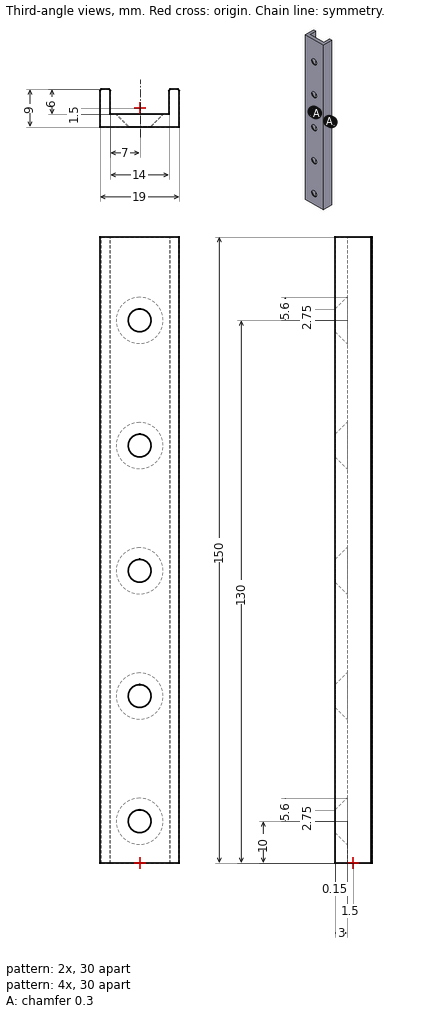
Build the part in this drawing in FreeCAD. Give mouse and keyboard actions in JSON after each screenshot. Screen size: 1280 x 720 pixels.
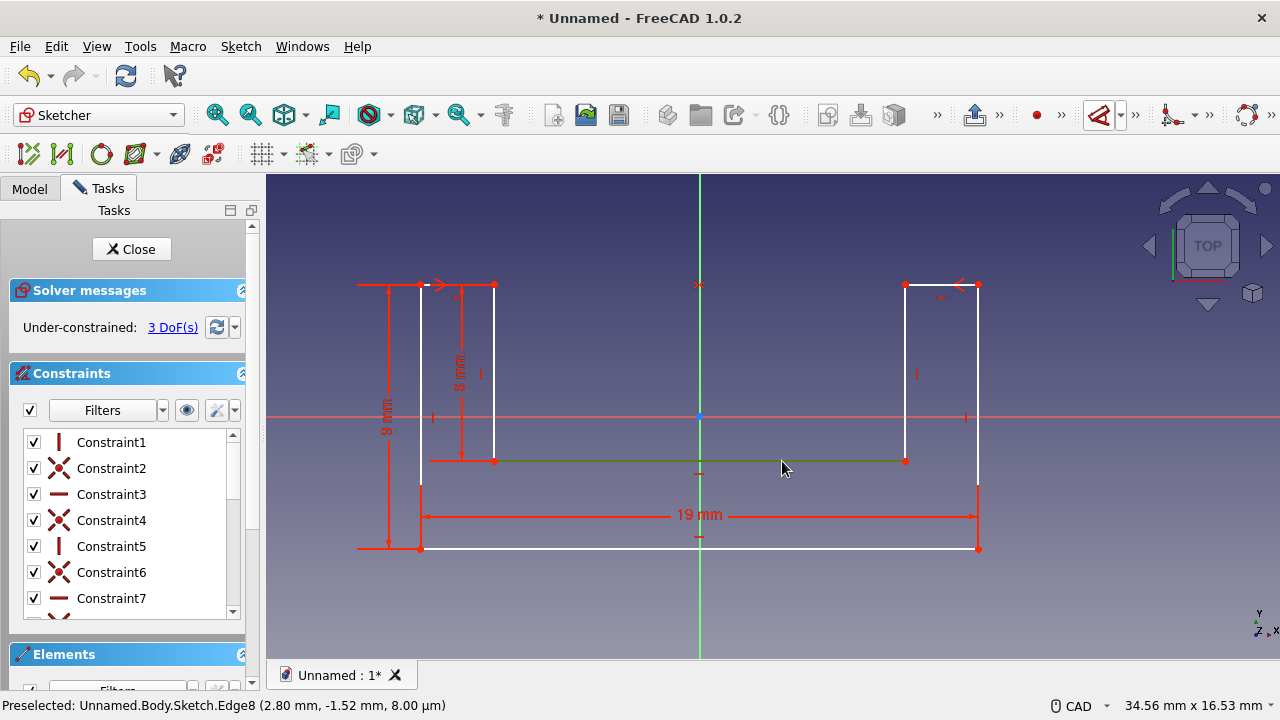
{"action": "left_click", "coordinate": [1120, 116]}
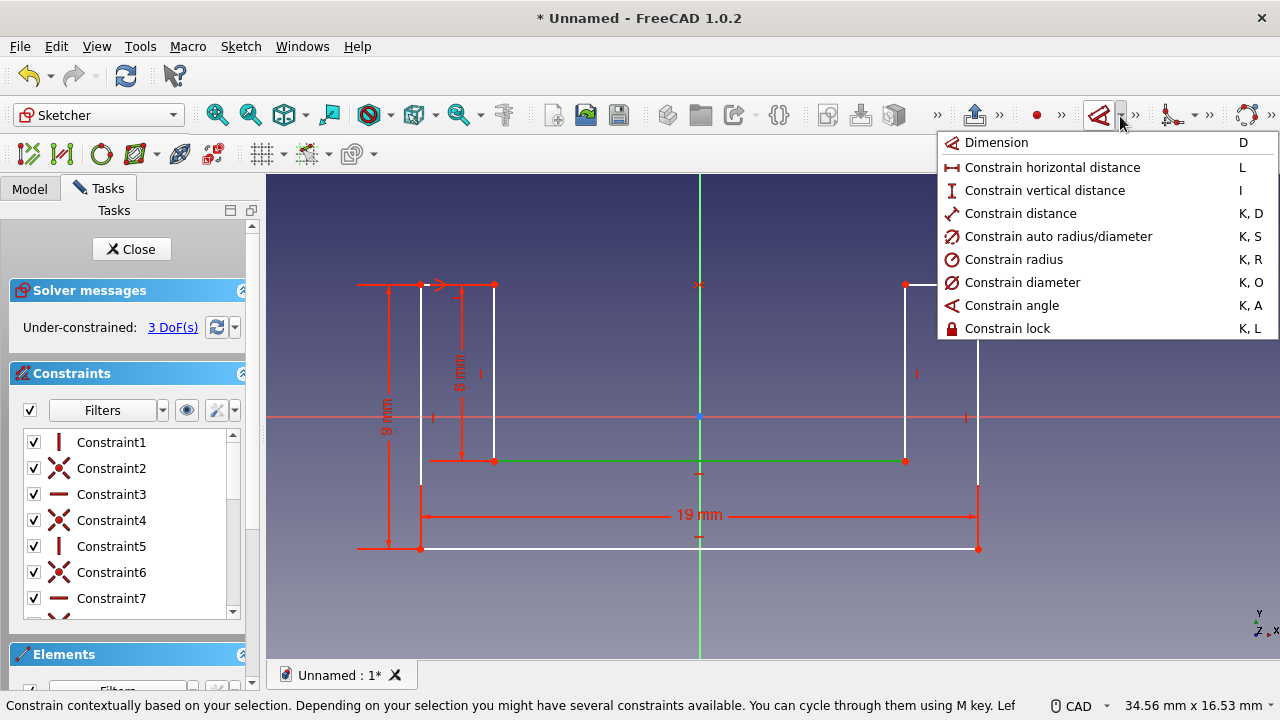
{"action": "left_click", "coordinate": [1108, 168]}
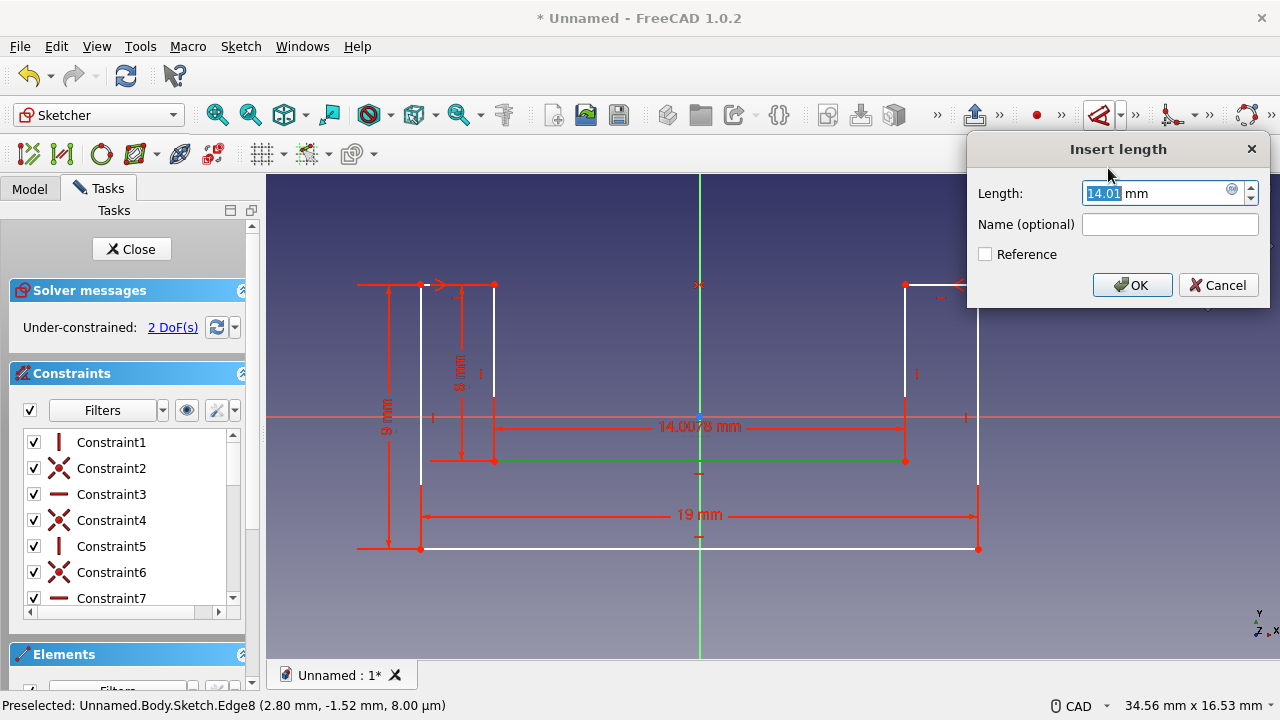
{"action": "type", "text": "14"}
{"action": "key", "text": "Return"}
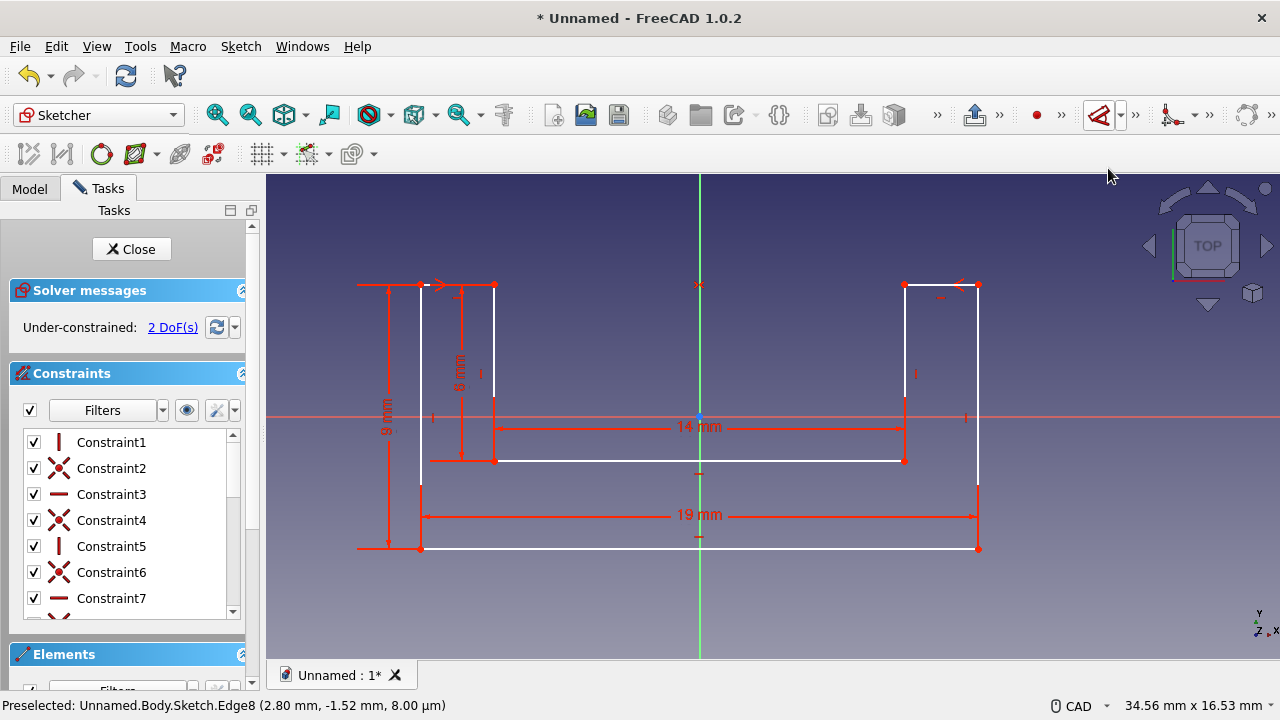
{"action": "left_click", "coordinate": [494, 461]}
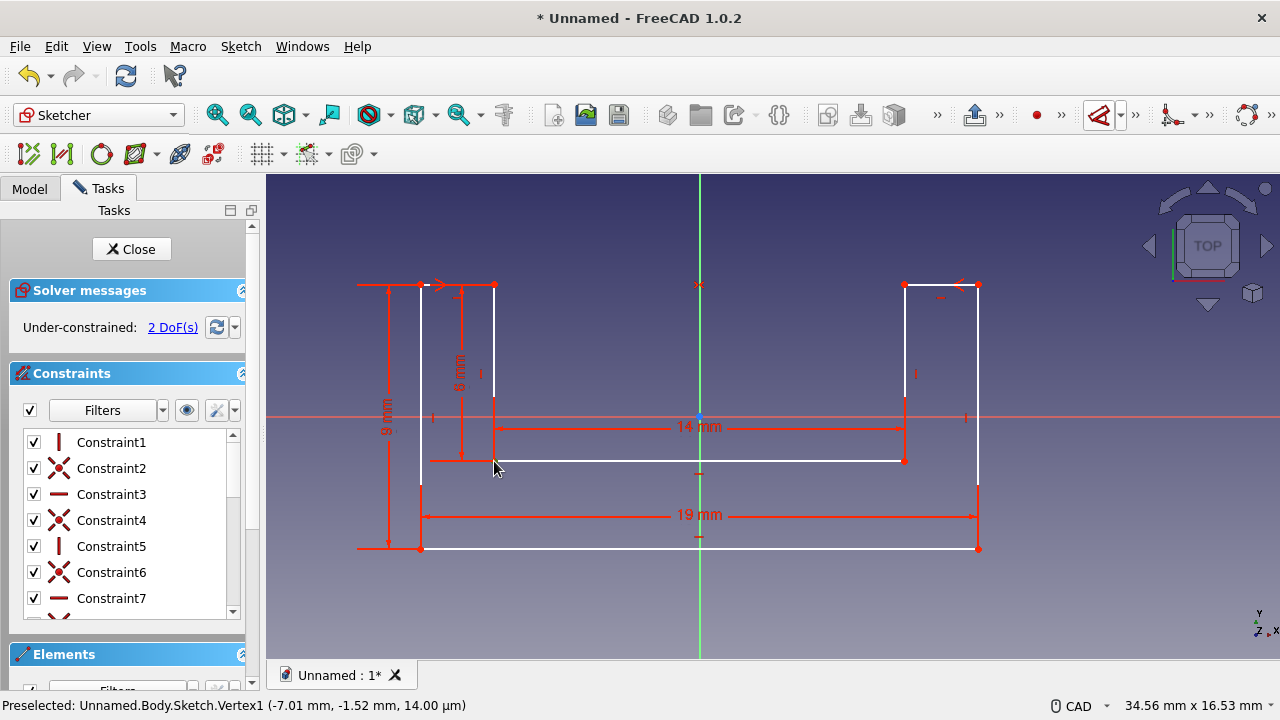
{"action": "left_click", "coordinate": [1120, 116]}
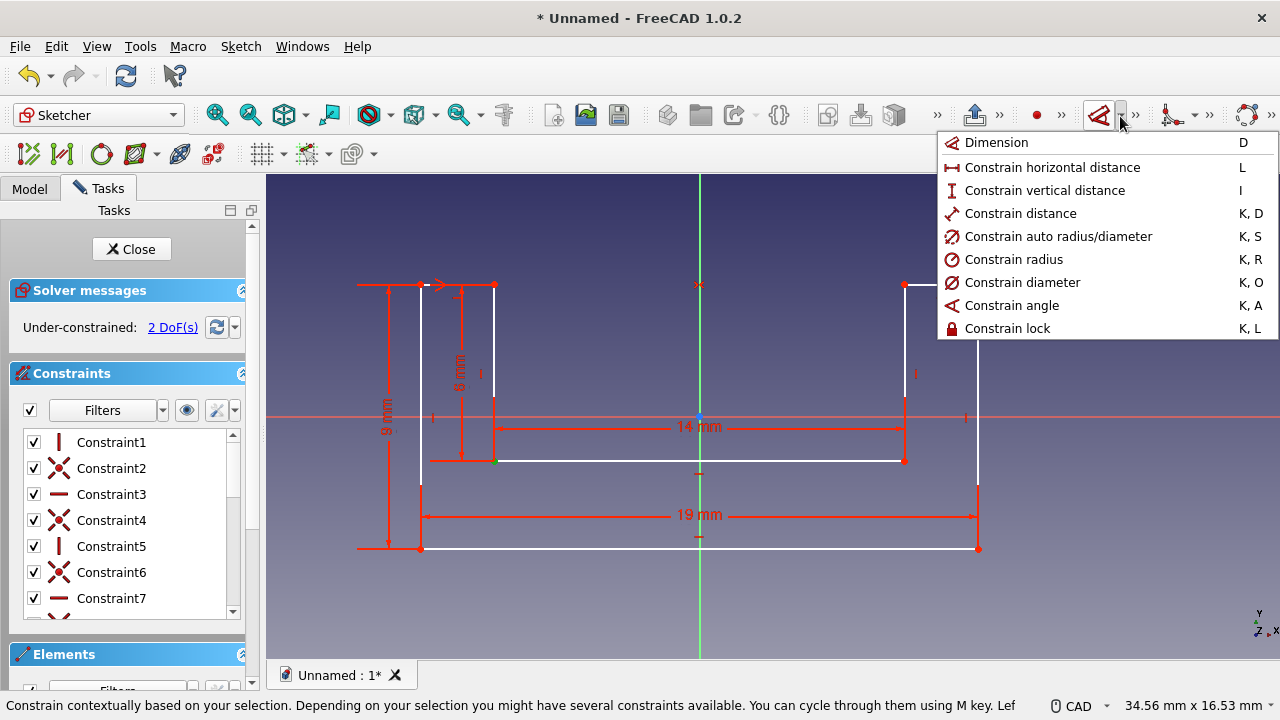
{"action": "left_click", "coordinate": [1108, 168]}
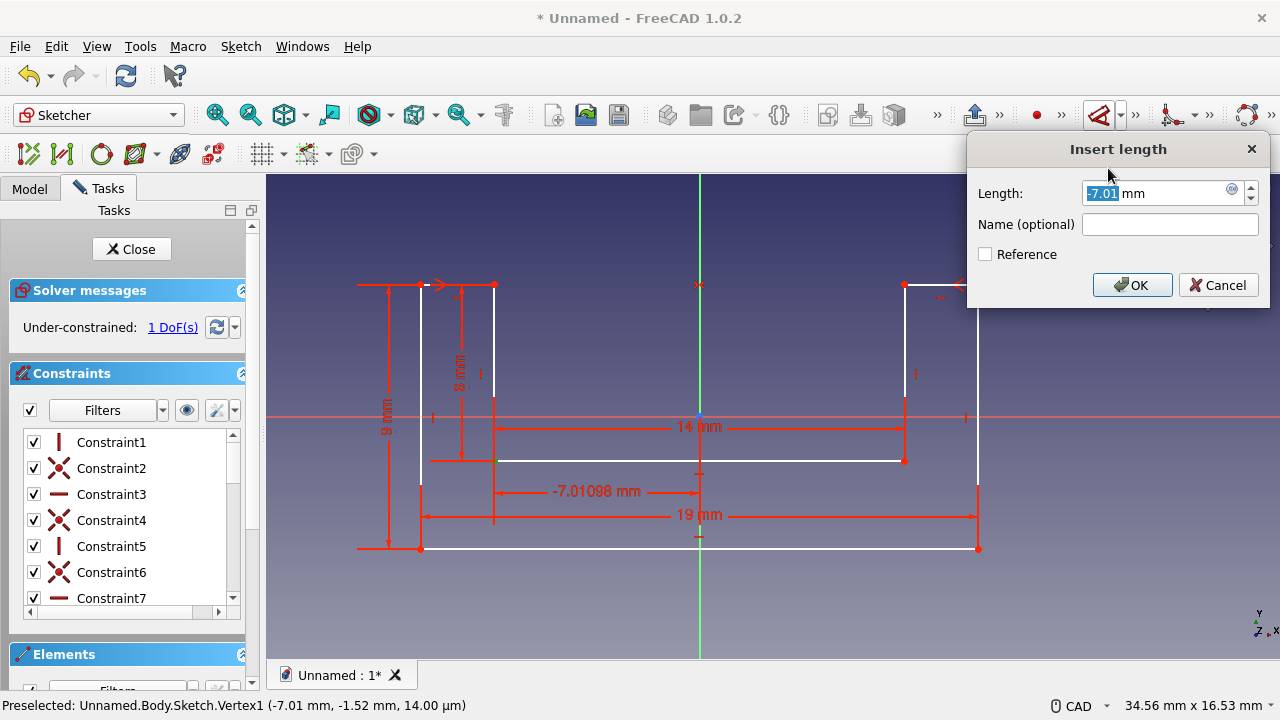
{"action": "type", "text": "-7"}
{"action": "key", "text": "Return"}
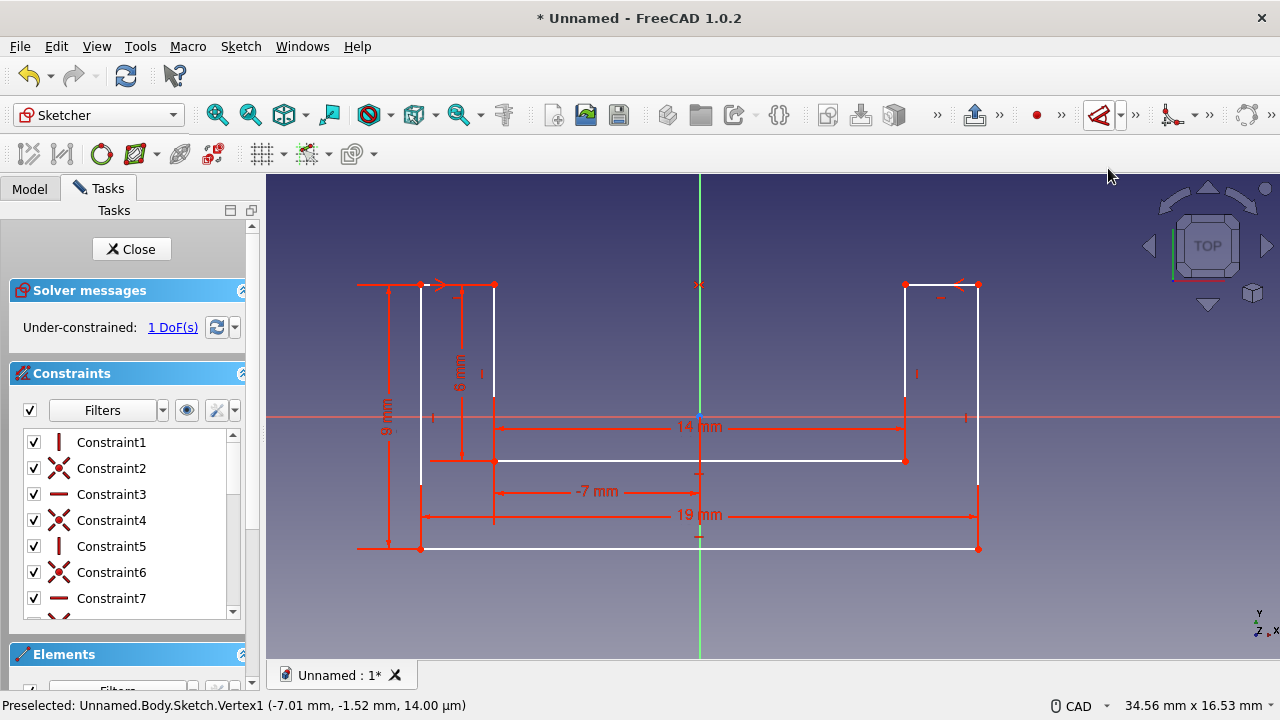
{"action": "left_click", "coordinate": [494, 461]}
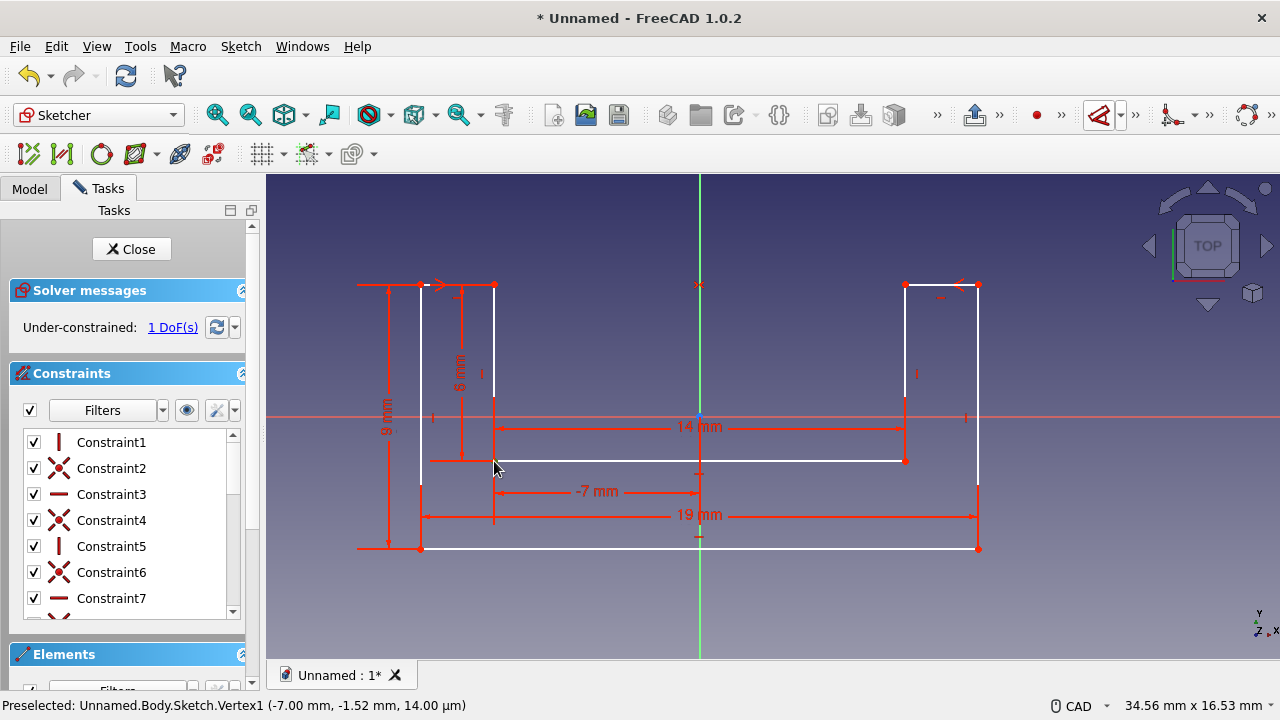
{"action": "left_click", "coordinate": [1120, 116]}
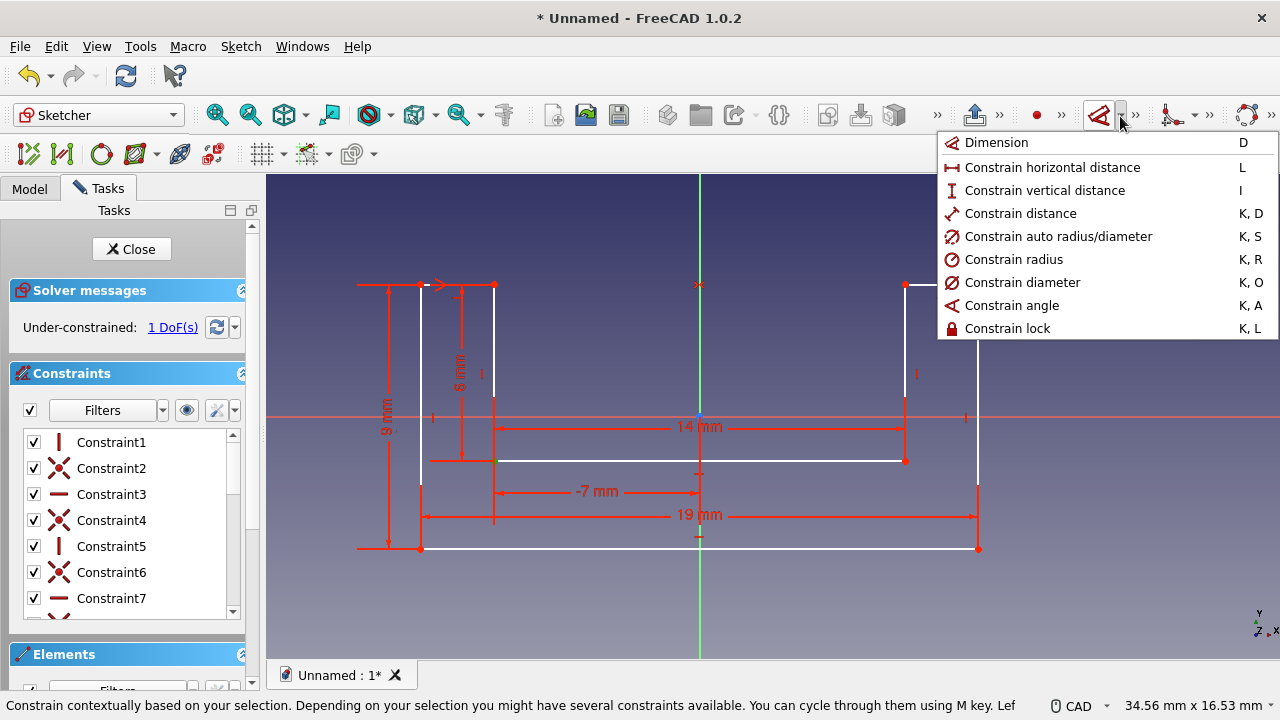
{"action": "left_click", "coordinate": [1108, 190]}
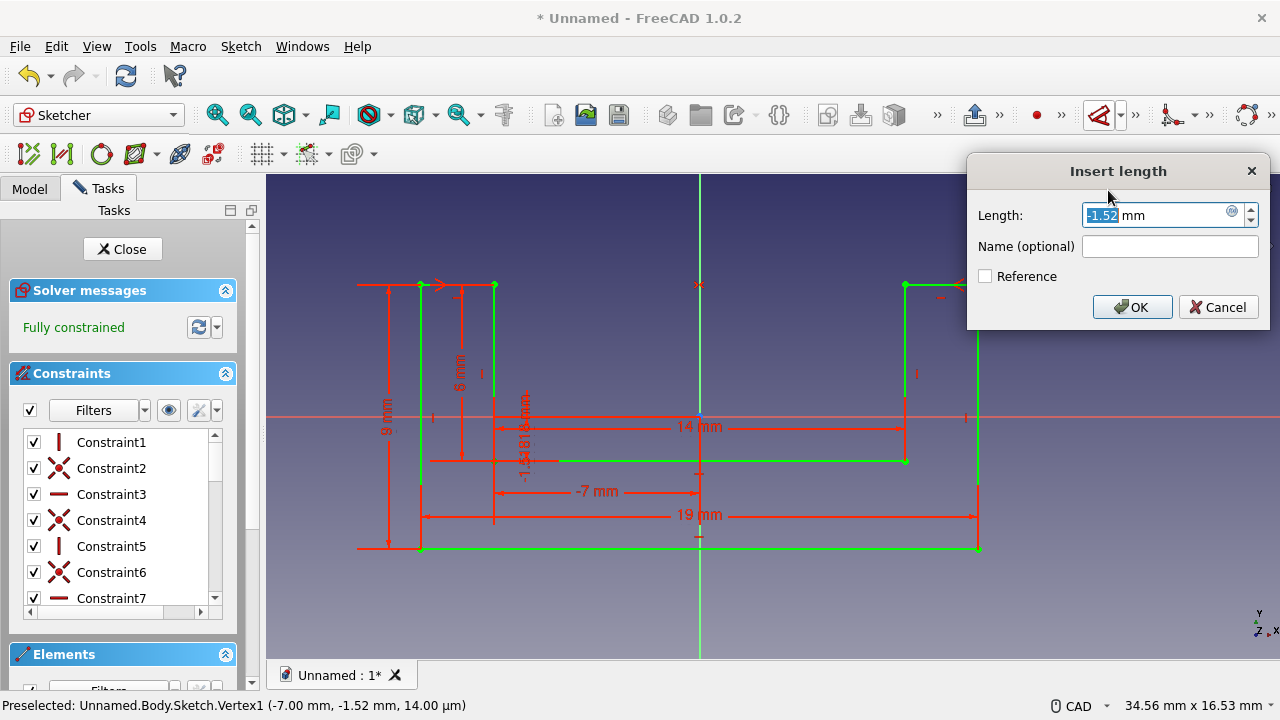
{"action": "type", "text": "-1.5"}
{"action": "key", "text": "Return"}